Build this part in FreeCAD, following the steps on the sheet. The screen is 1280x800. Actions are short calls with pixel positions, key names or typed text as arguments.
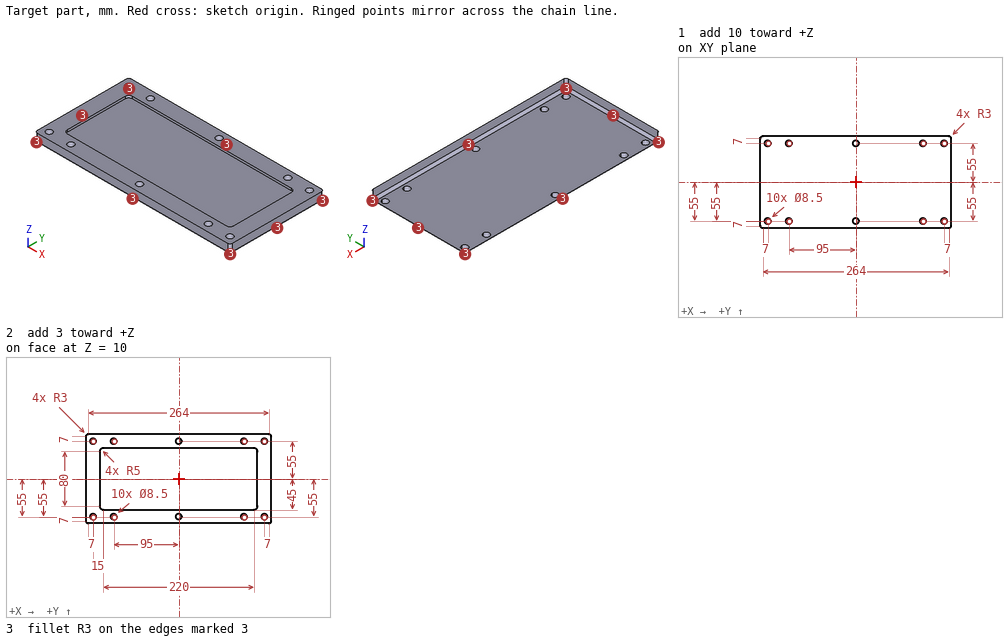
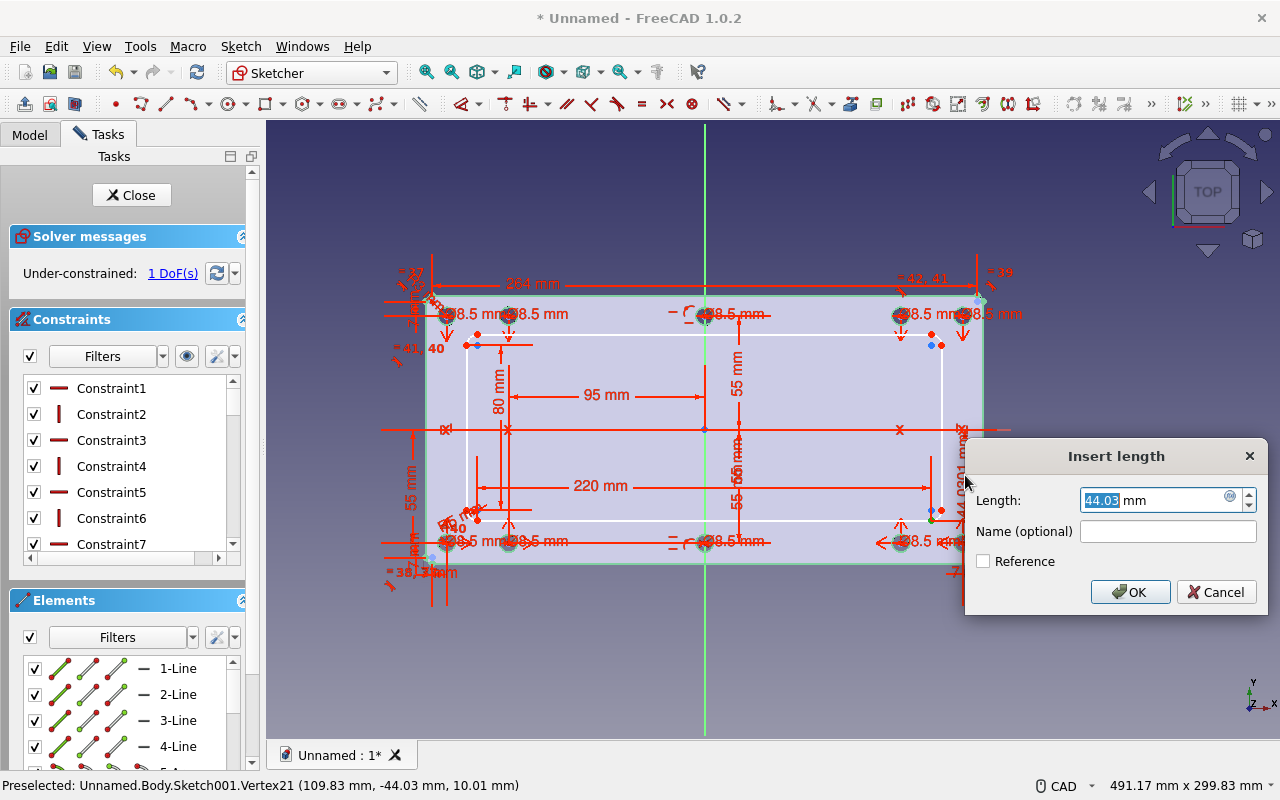
text(45)
key(Return)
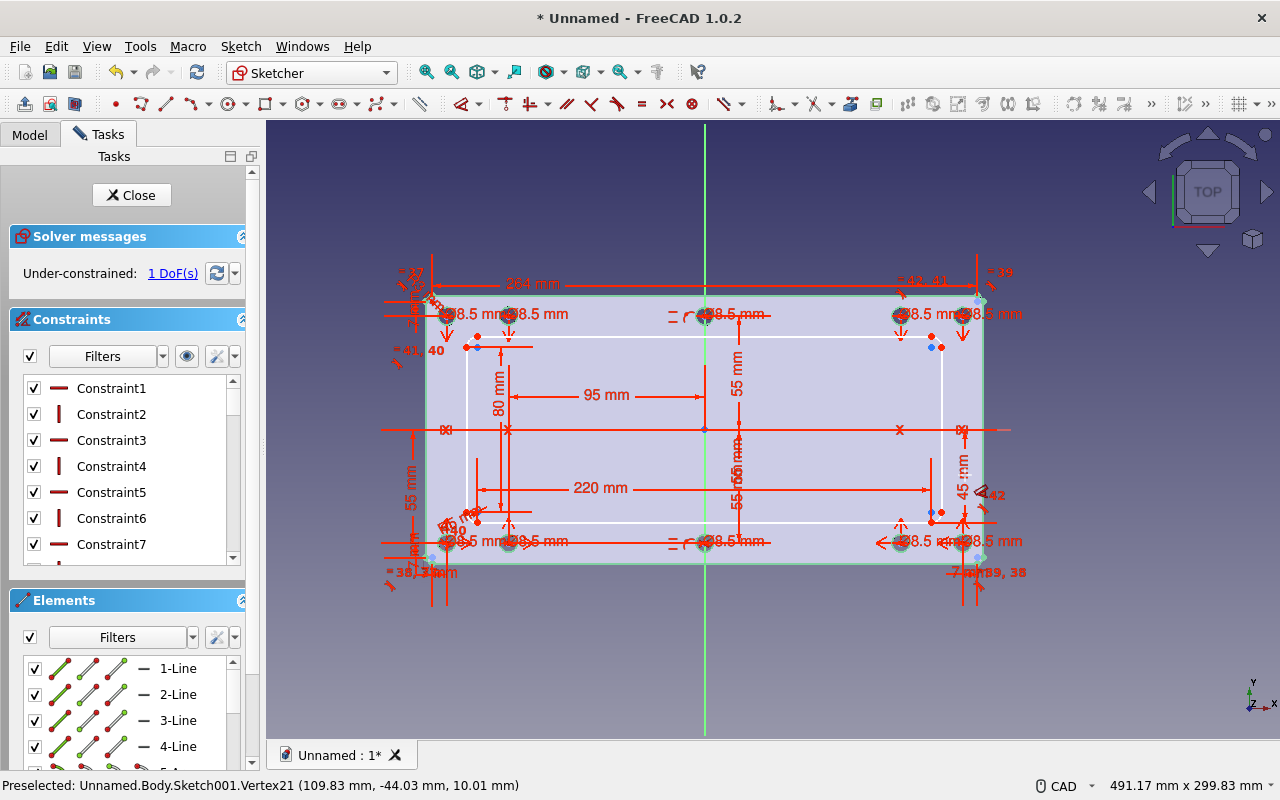
scroll(477, 523, up, 2)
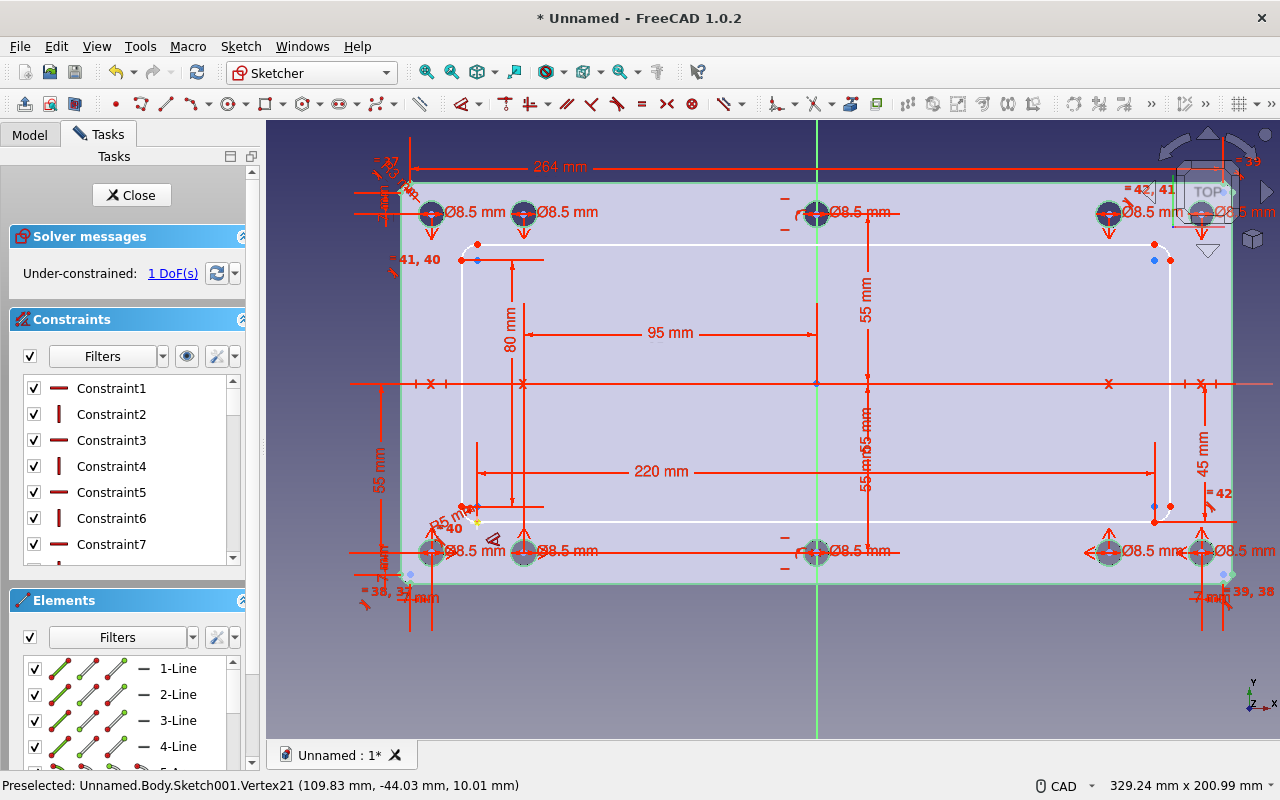
click(477, 522)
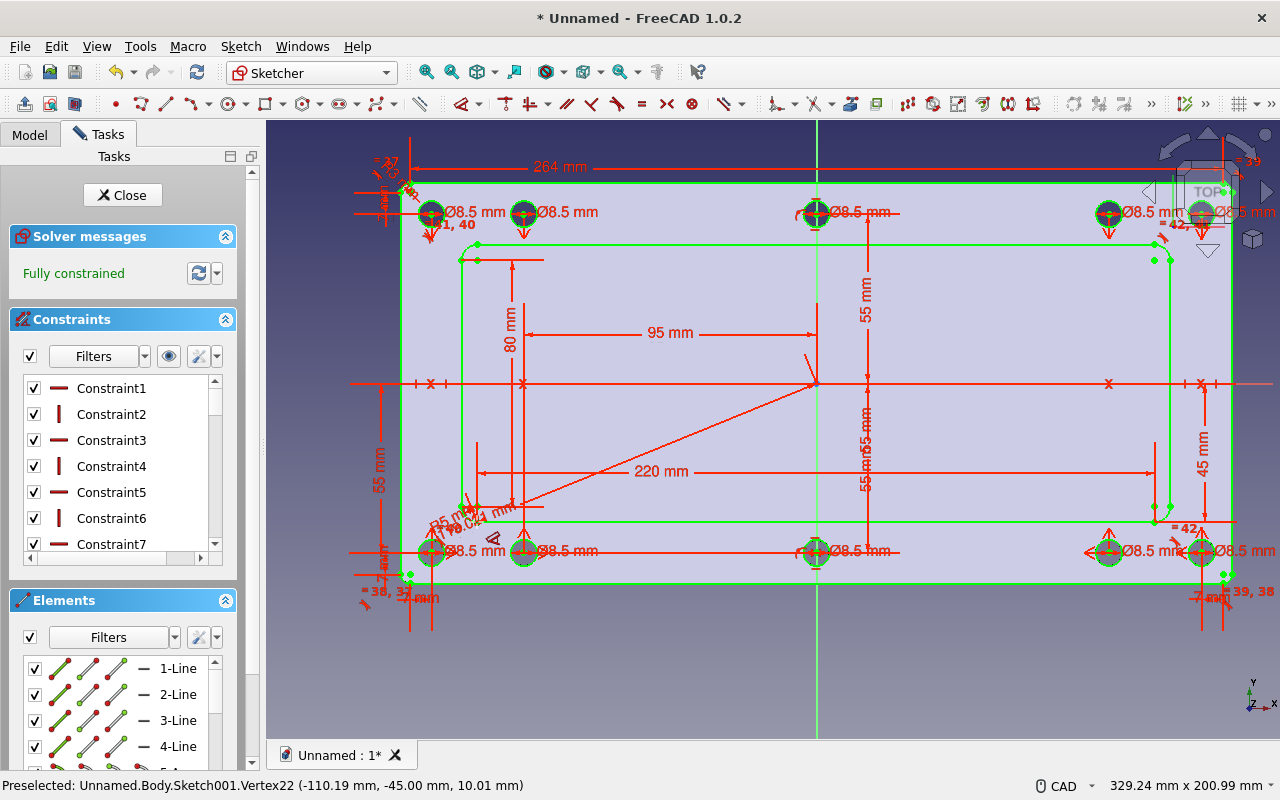
click(432, 553)
click(454, 635)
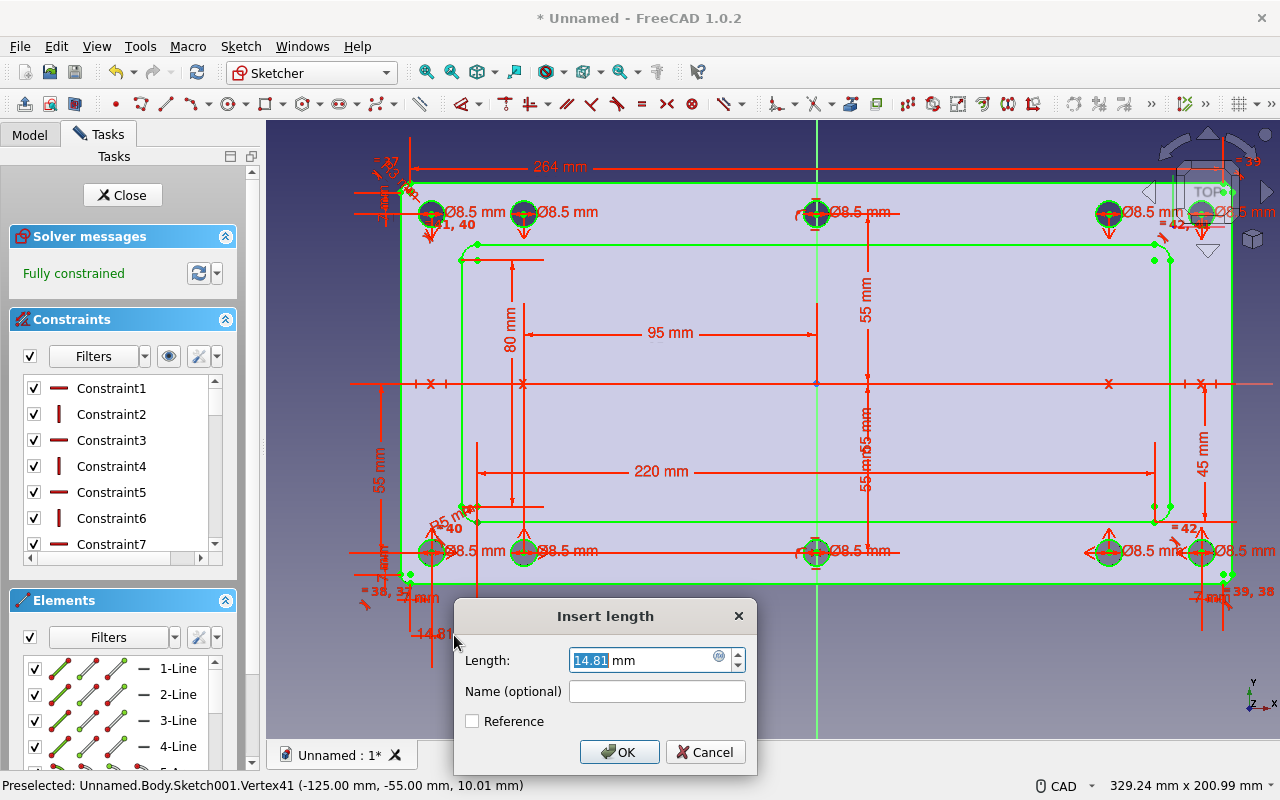
text(15)
key(Return)
key(Escape)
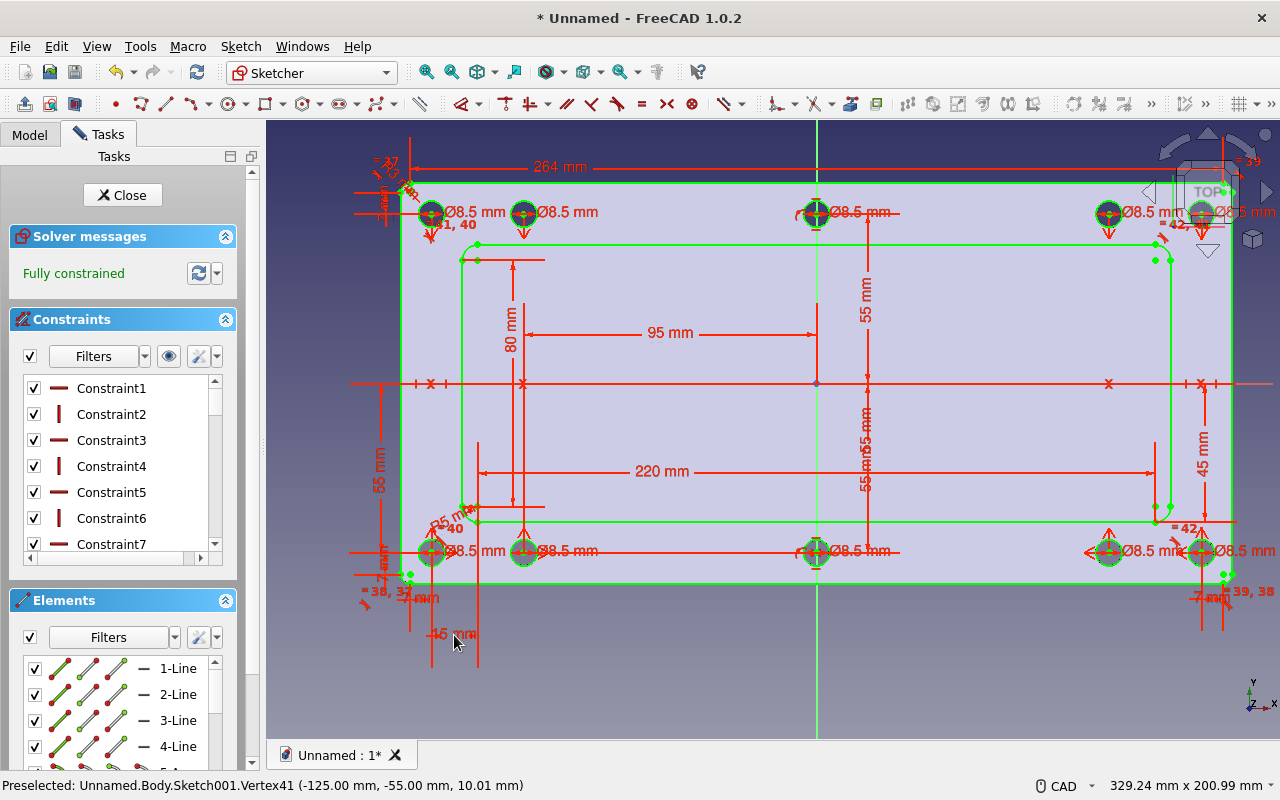
click(123, 195)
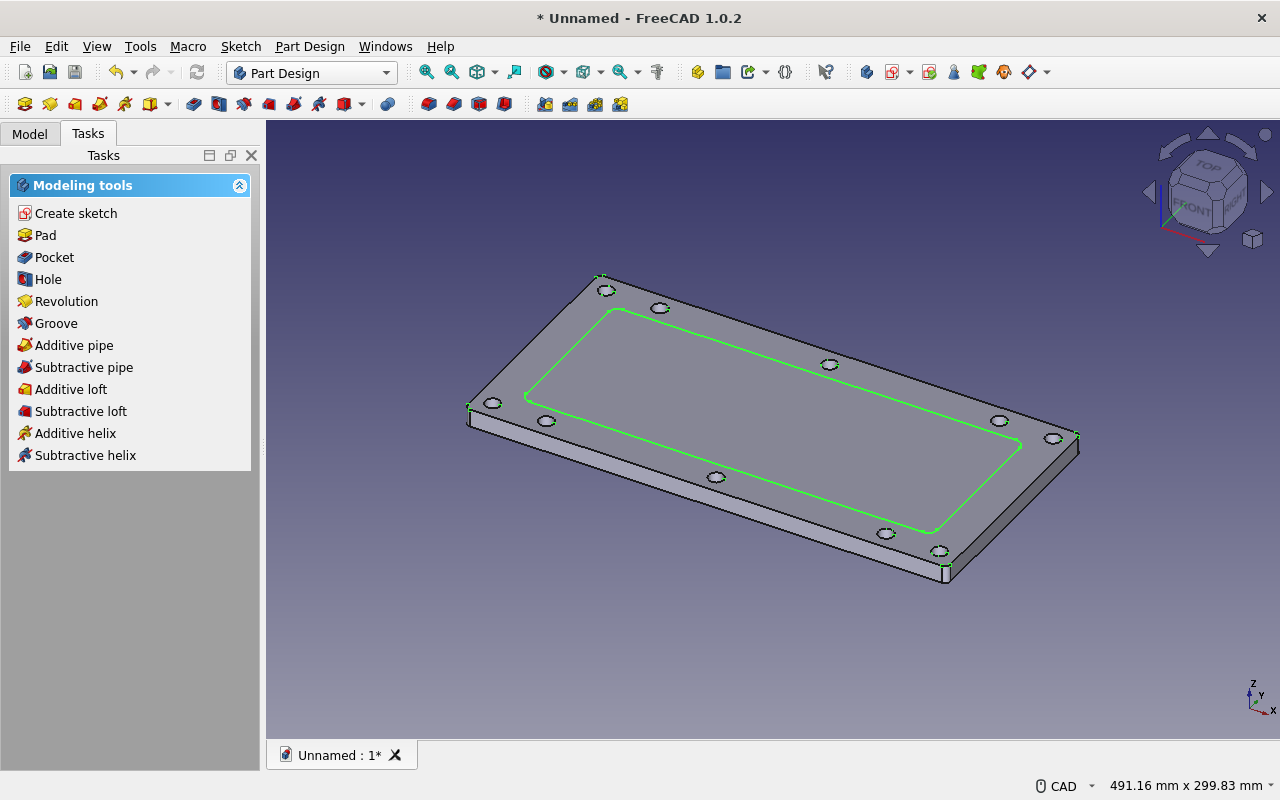
click(25, 104)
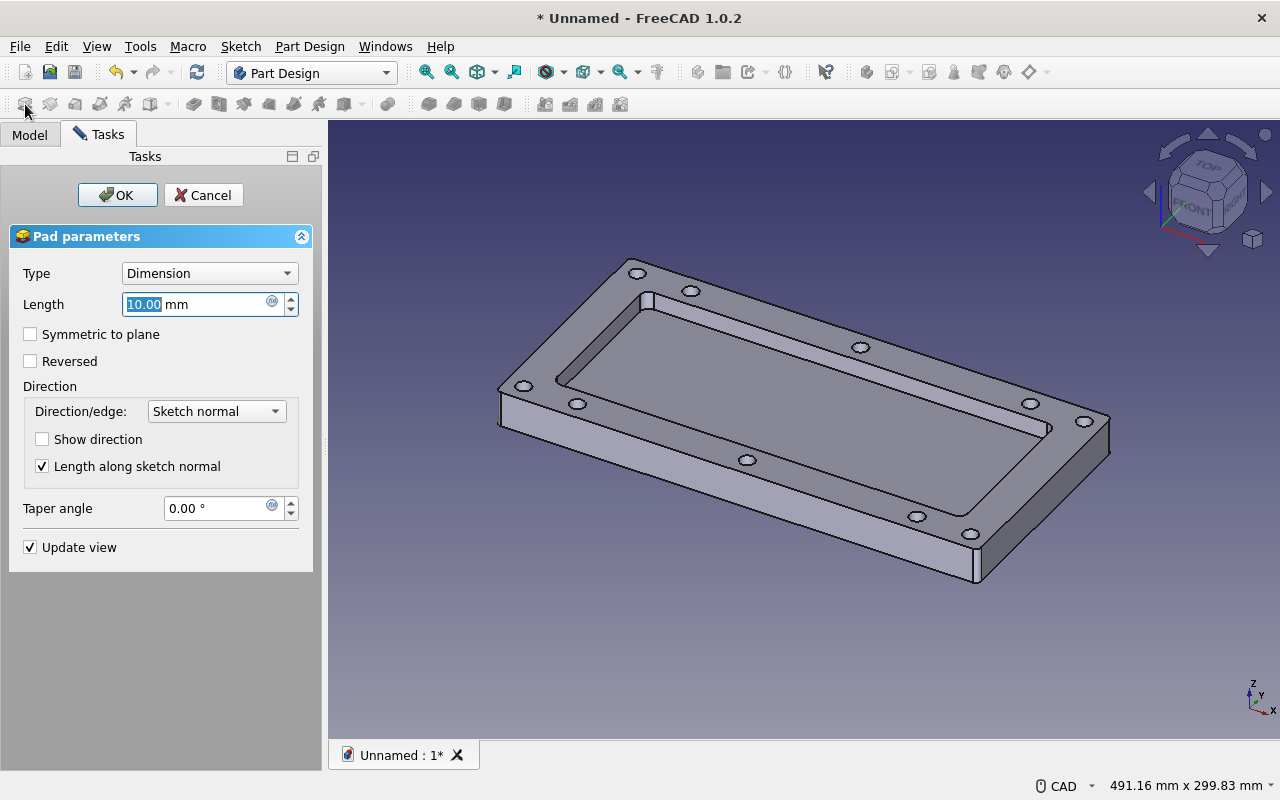
text(3)
key(Tab)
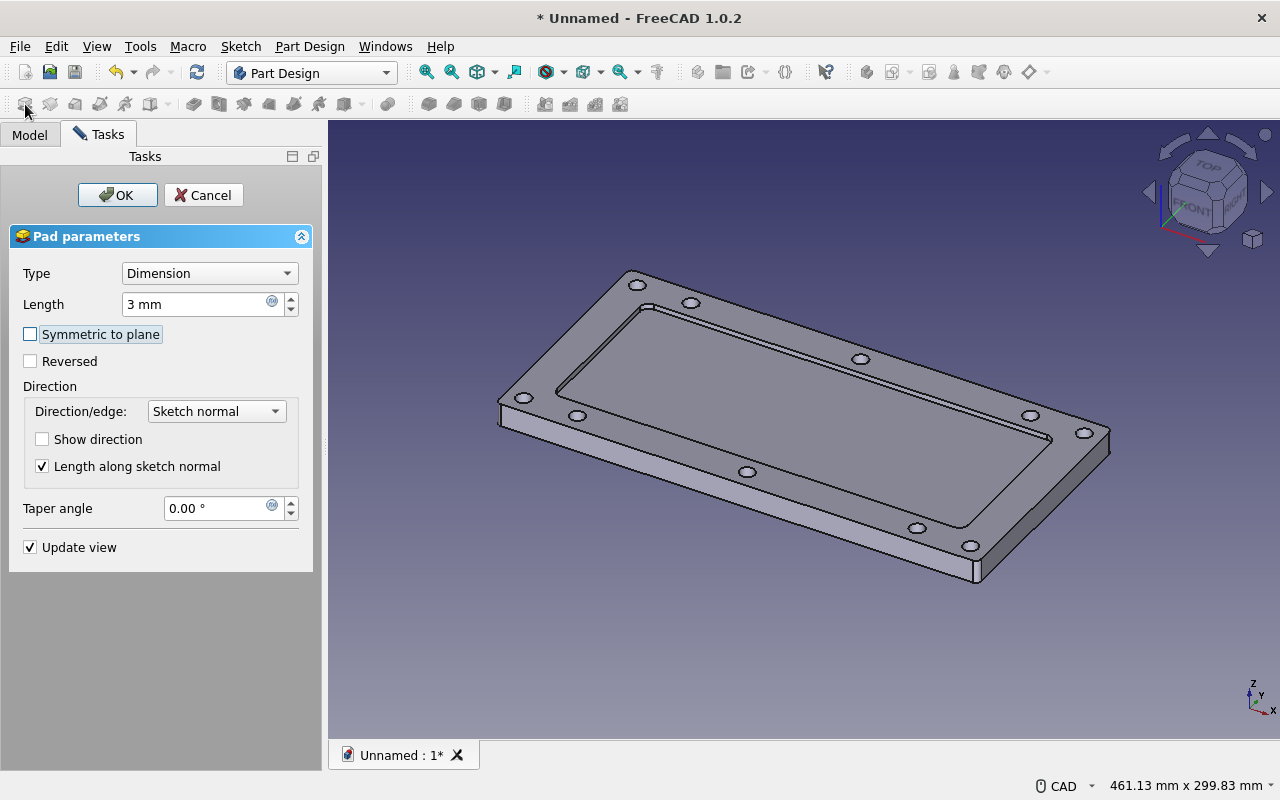
click(118, 195)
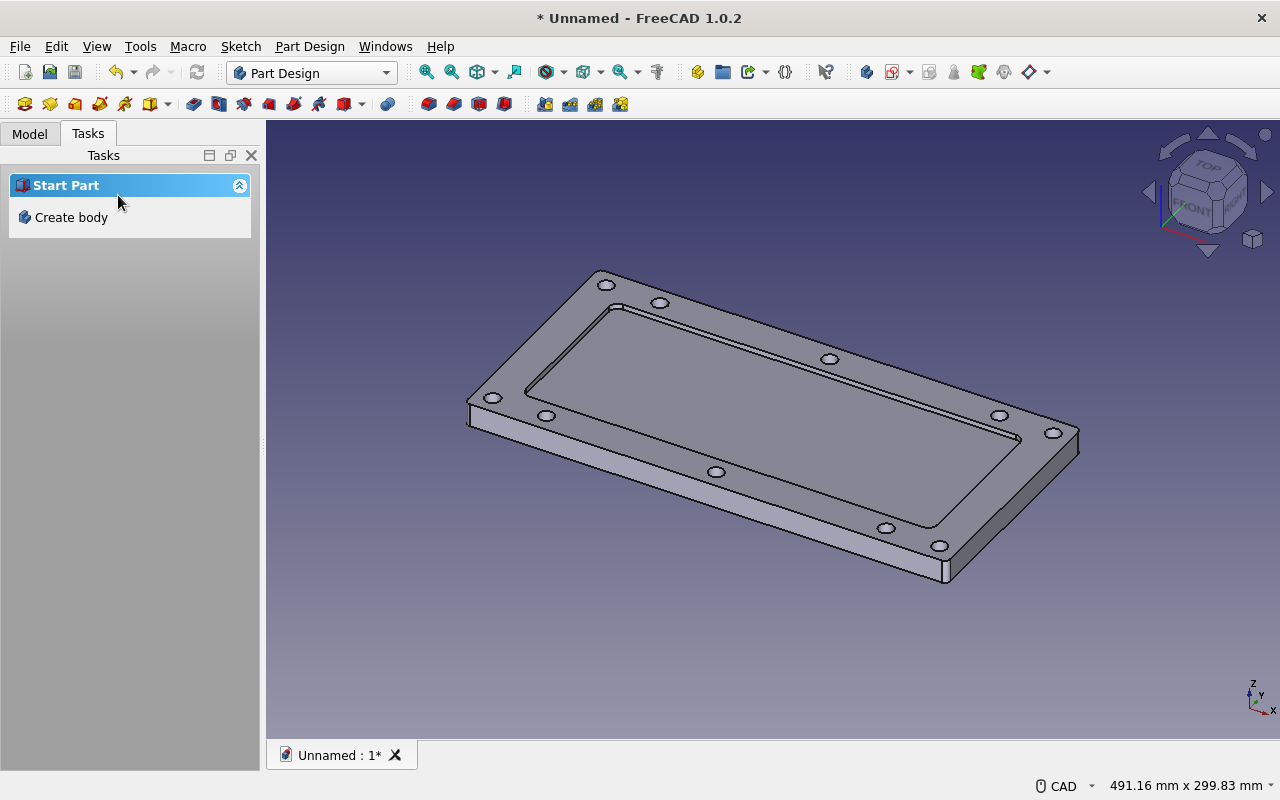
click(950, 581)